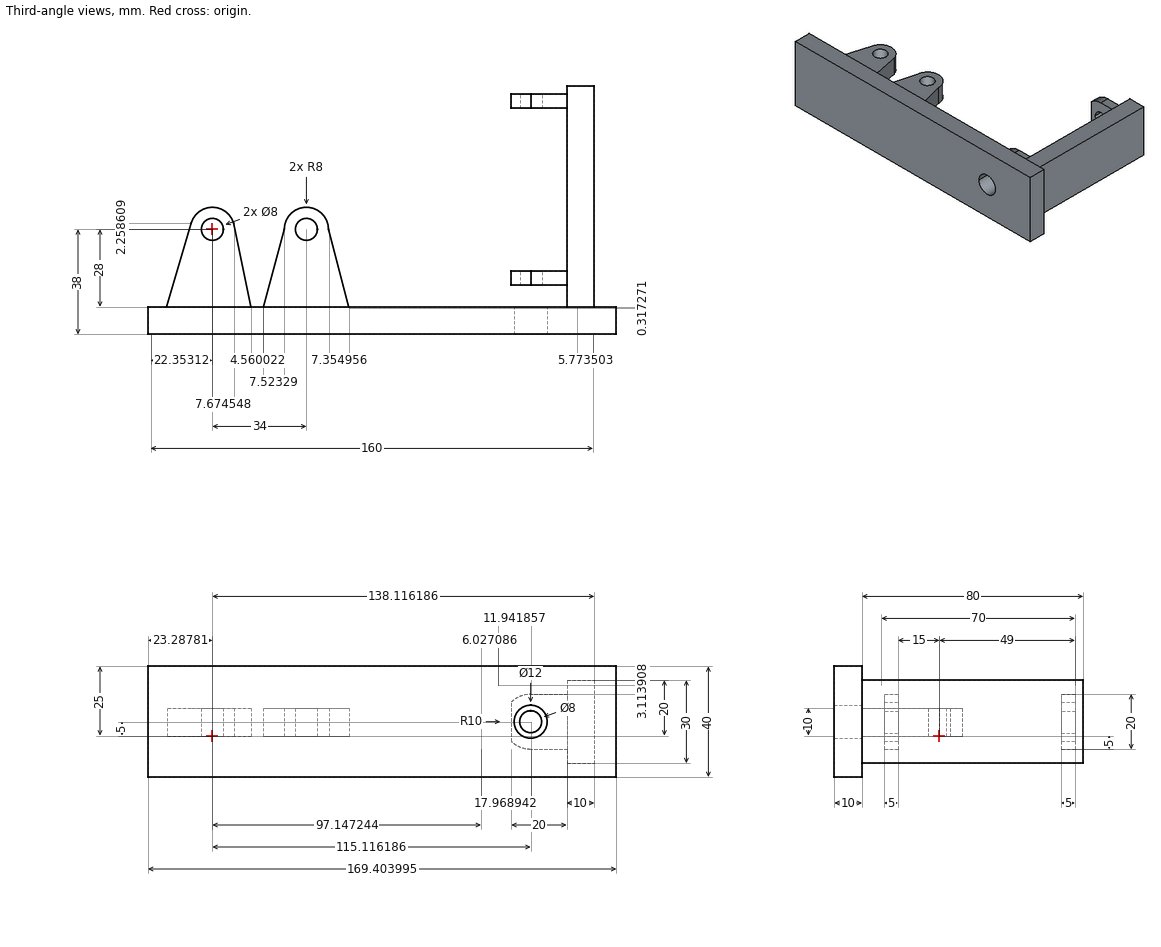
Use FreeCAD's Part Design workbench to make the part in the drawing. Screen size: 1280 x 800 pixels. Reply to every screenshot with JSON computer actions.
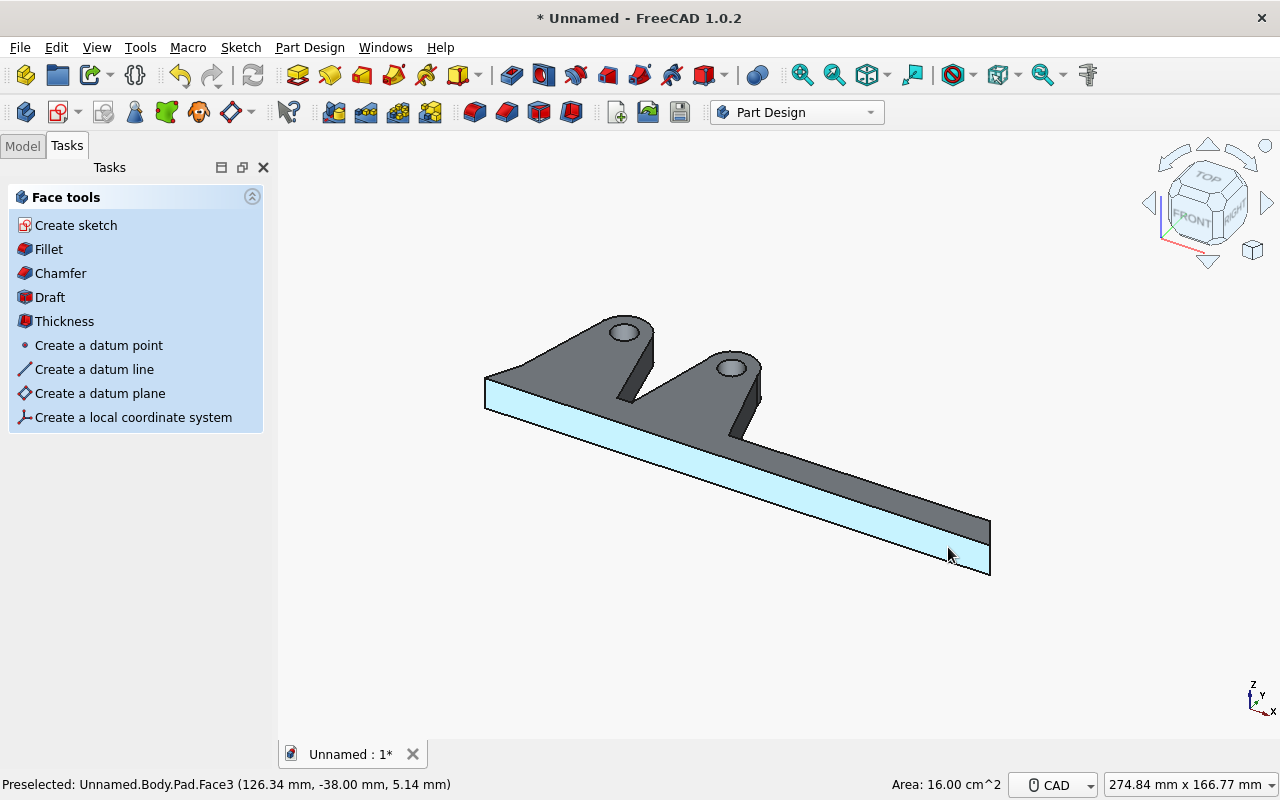
{"action": "left_click", "coordinate": [58, 112]}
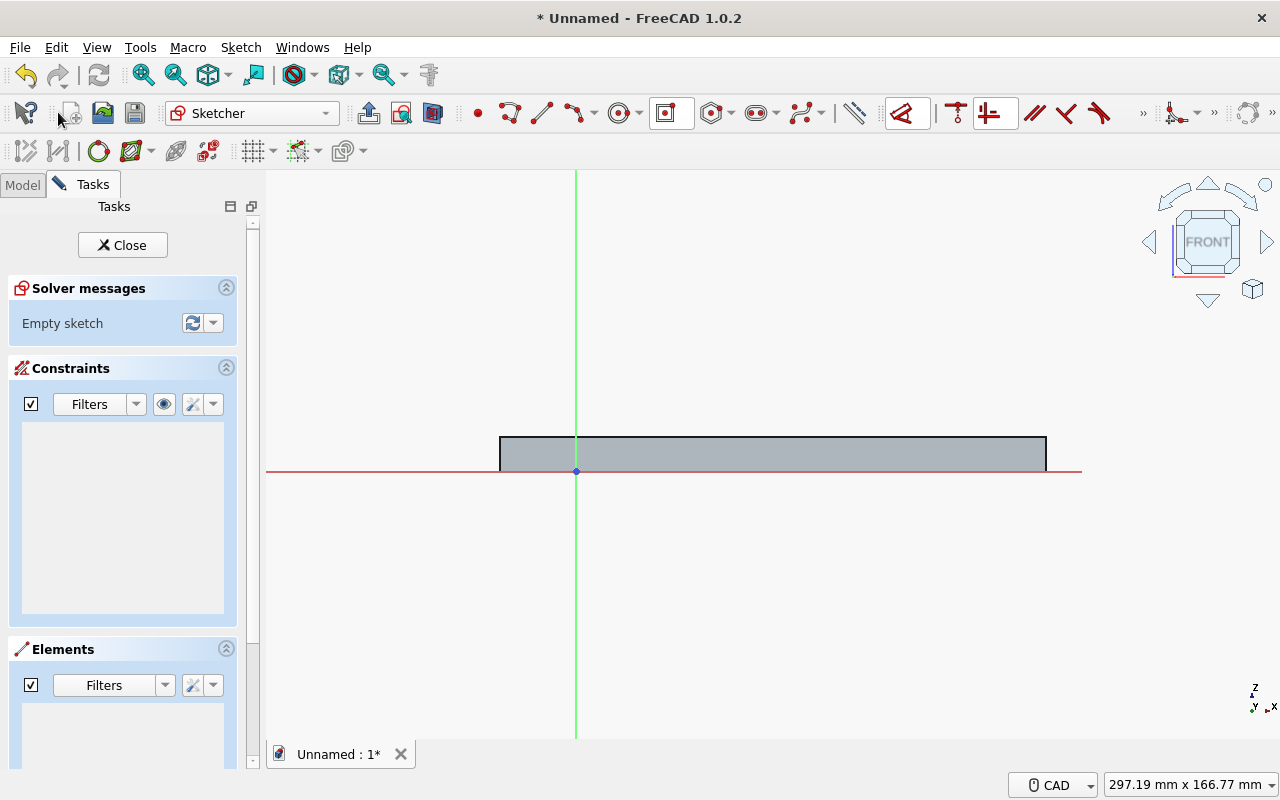
{"action": "left_click", "coordinate": [688, 114]}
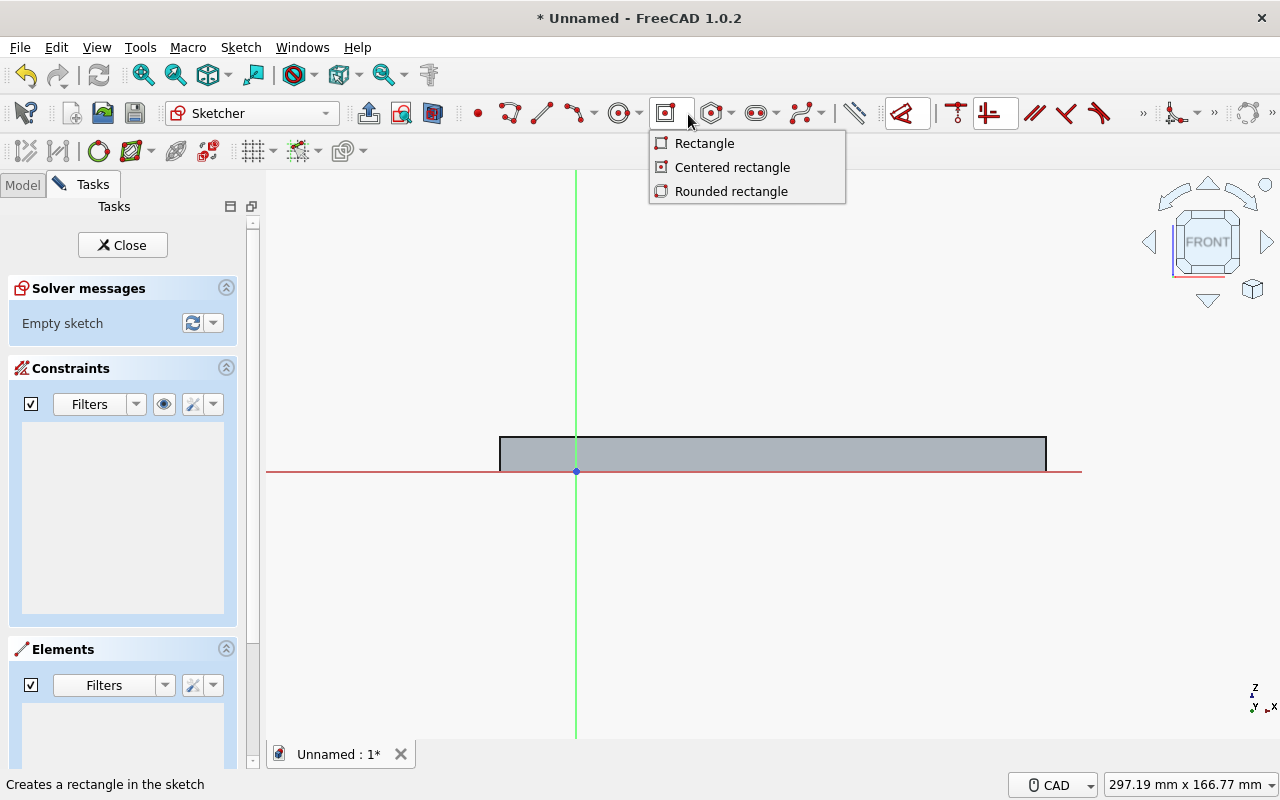
{"action": "left_click", "coordinate": [748, 143]}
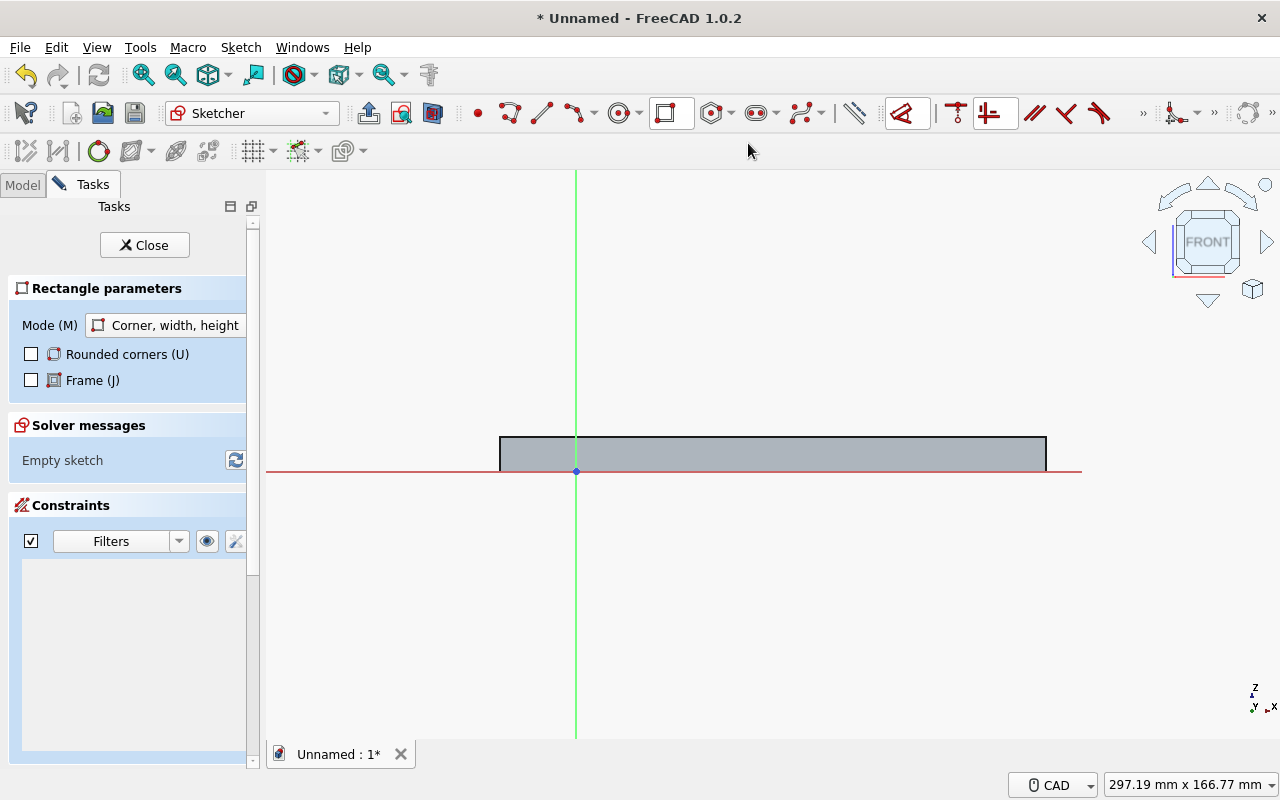
{"action": "left_click", "coordinate": [497, 386]}
{"action": "mouse_move", "coordinate": [1075, 523]}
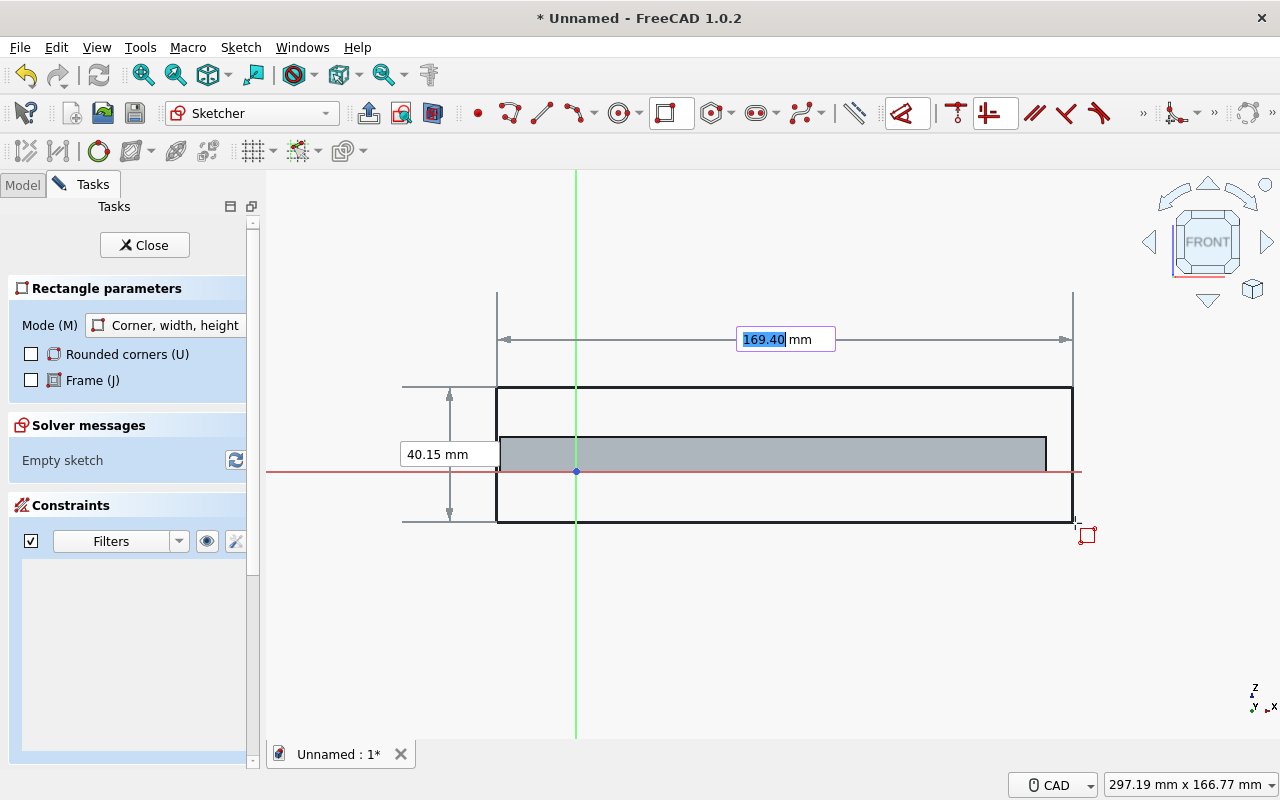
{"action": "type", "text": "169.403995"}
{"action": "key", "text": "Tab"}
{"action": "type", "text": "40"}
{"action": "key", "text": "Return"}
{"action": "key", "text": "Escape"}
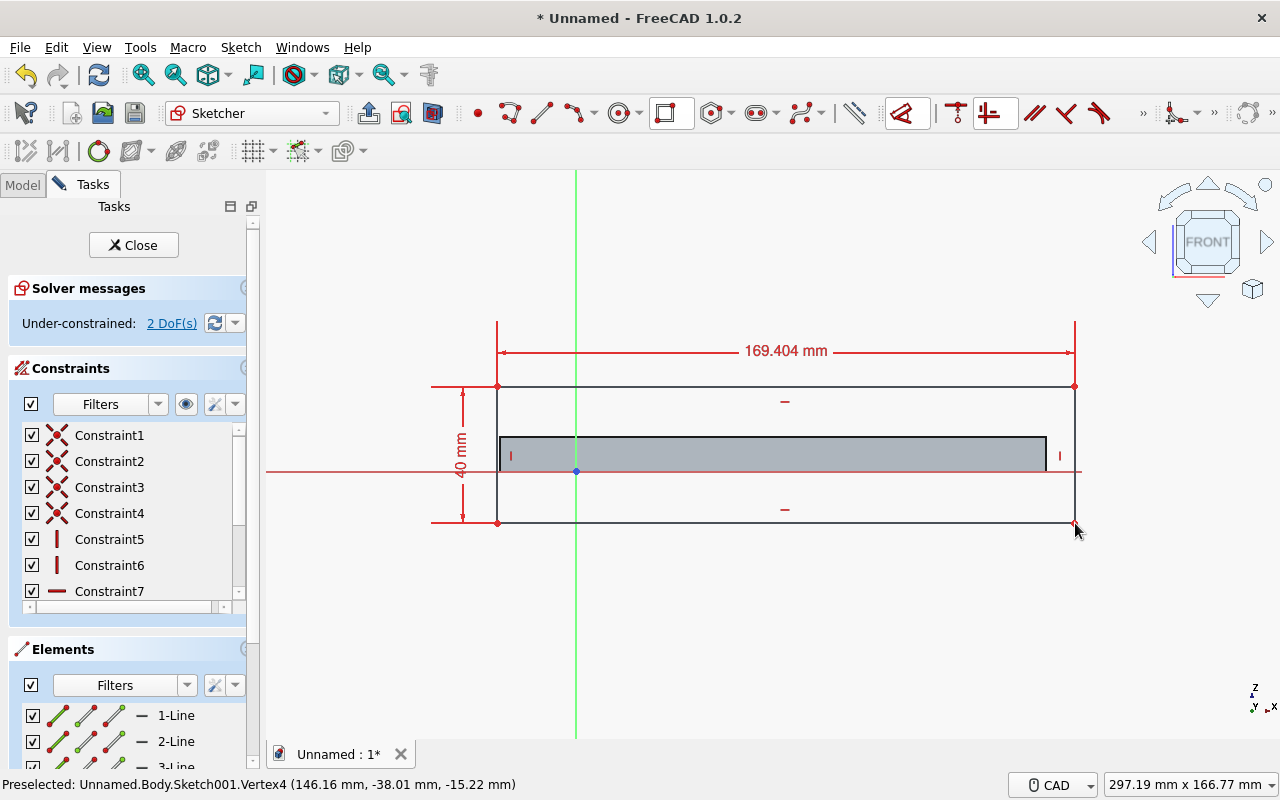
{"action": "left_click", "coordinate": [497, 387]}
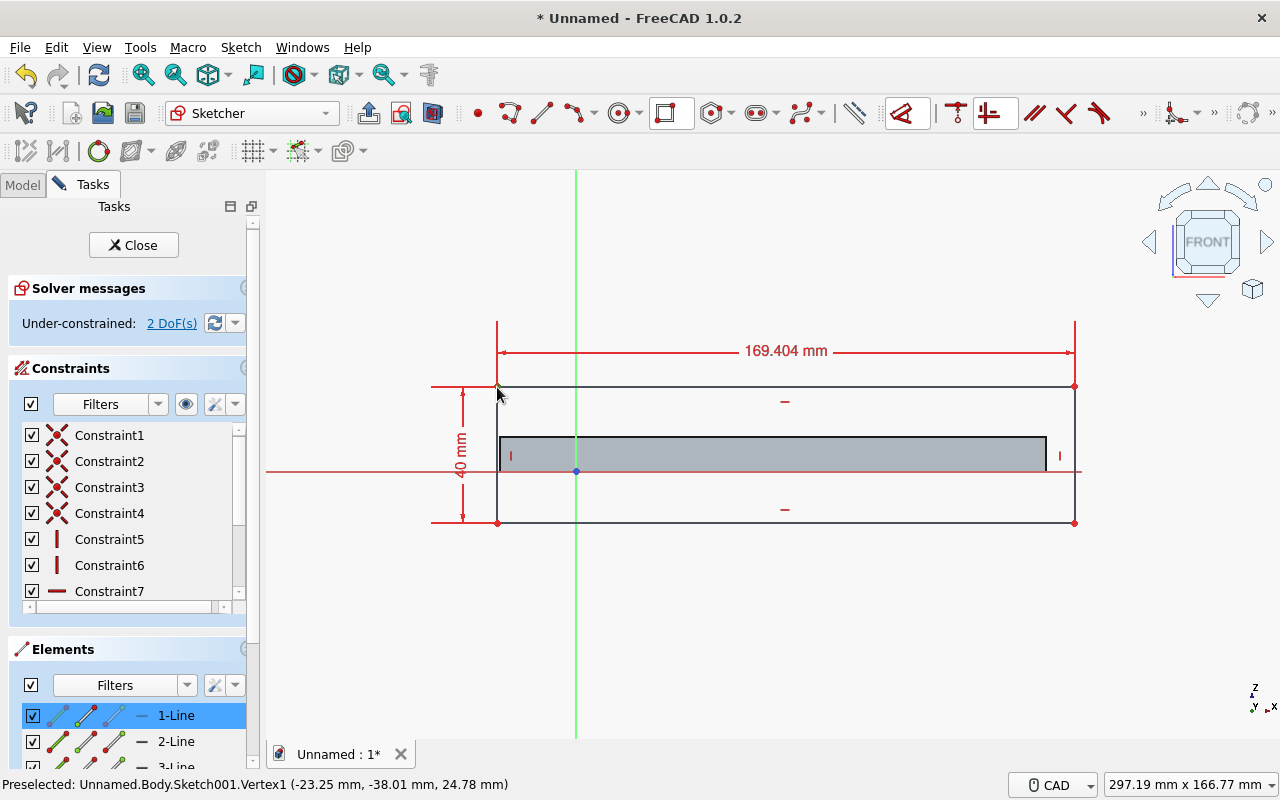
{"action": "key", "text": "i"}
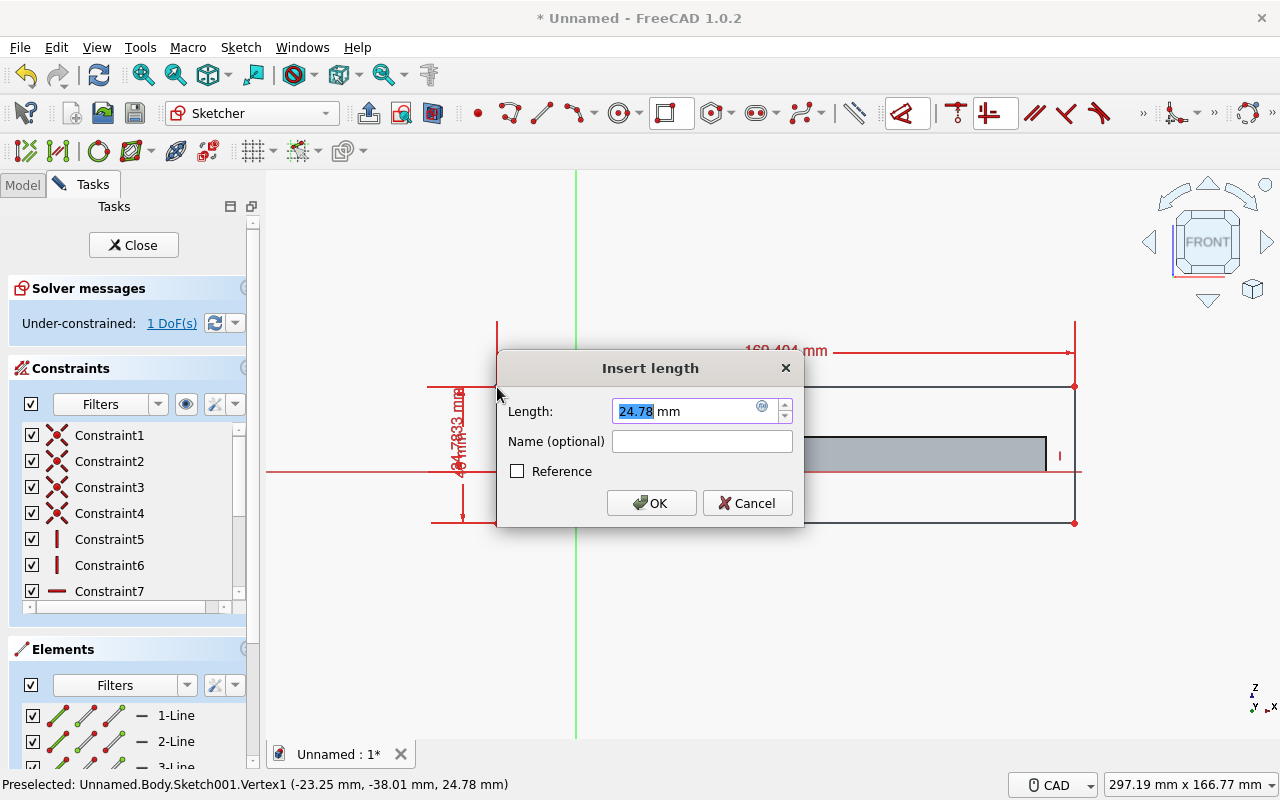
{"action": "type", "text": "25"}
{"action": "key", "text": "Return"}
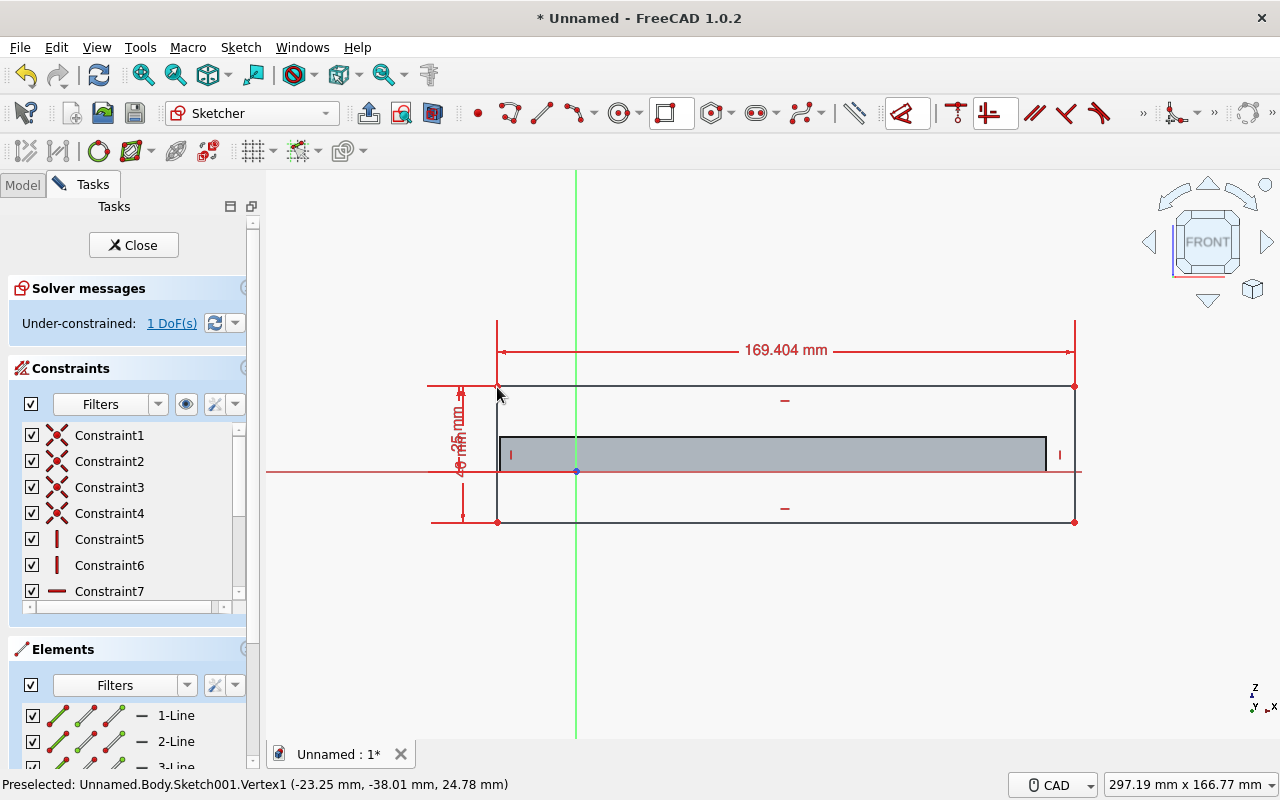
{"action": "left_click", "coordinate": [497, 386]}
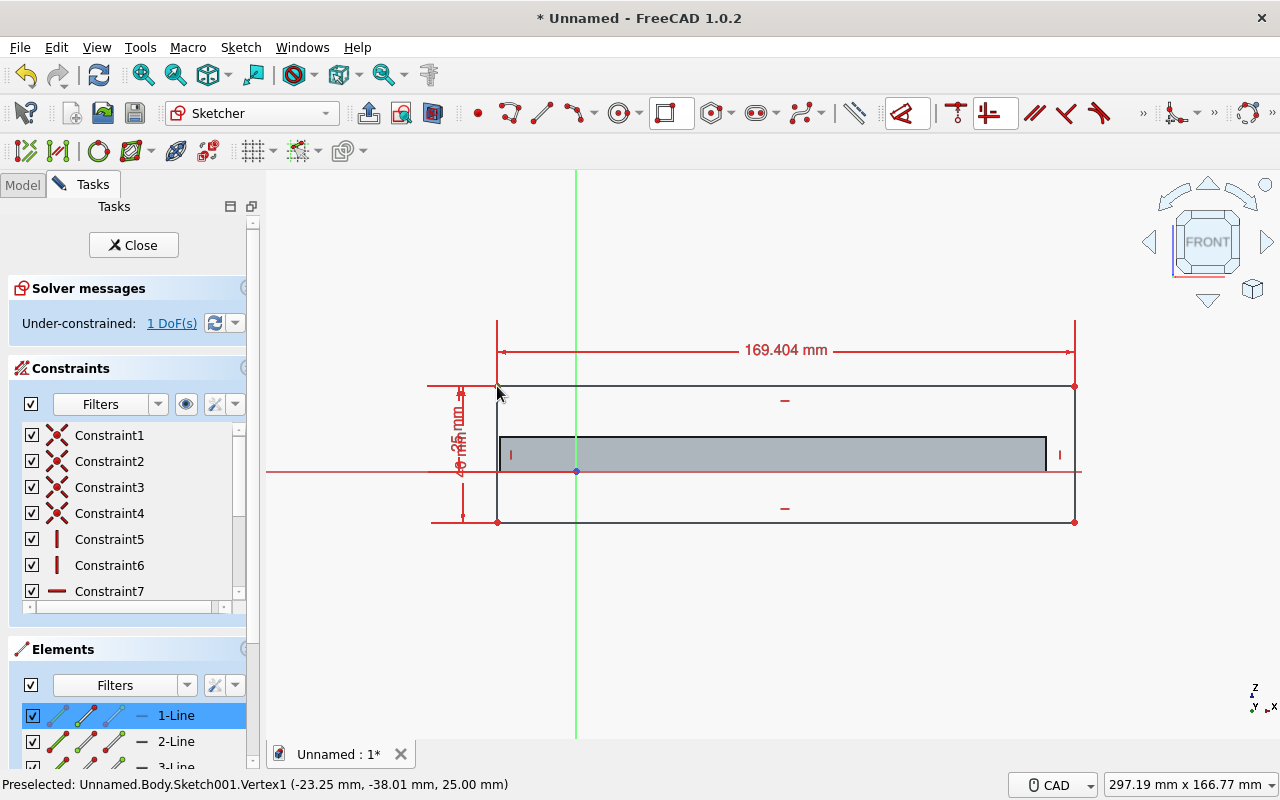
{"action": "left_click", "coordinate": [924, 114]}